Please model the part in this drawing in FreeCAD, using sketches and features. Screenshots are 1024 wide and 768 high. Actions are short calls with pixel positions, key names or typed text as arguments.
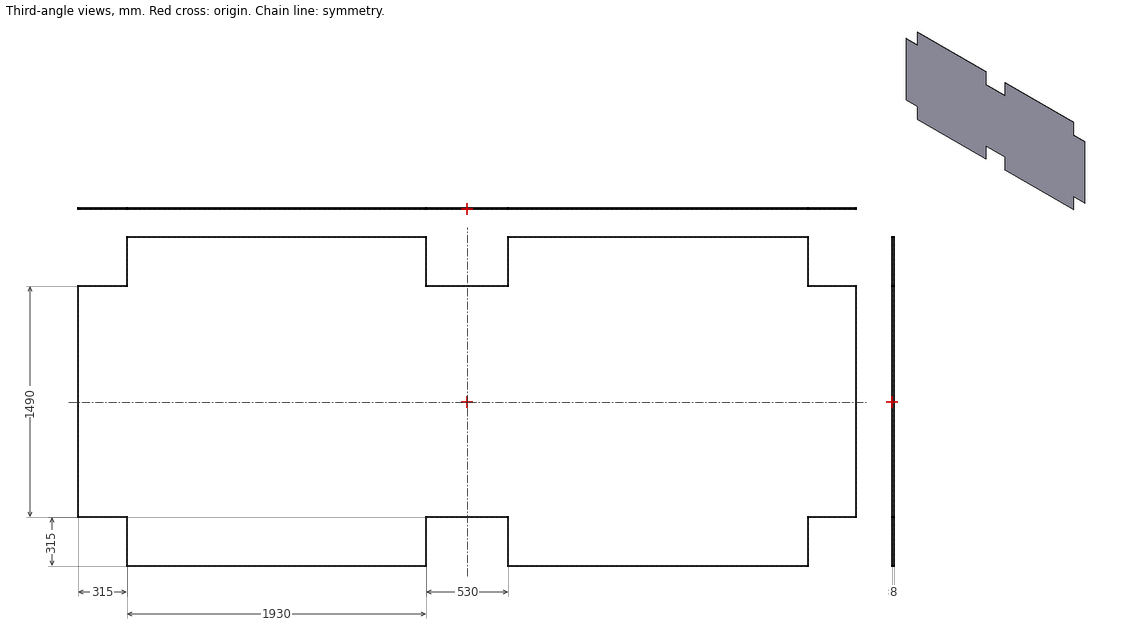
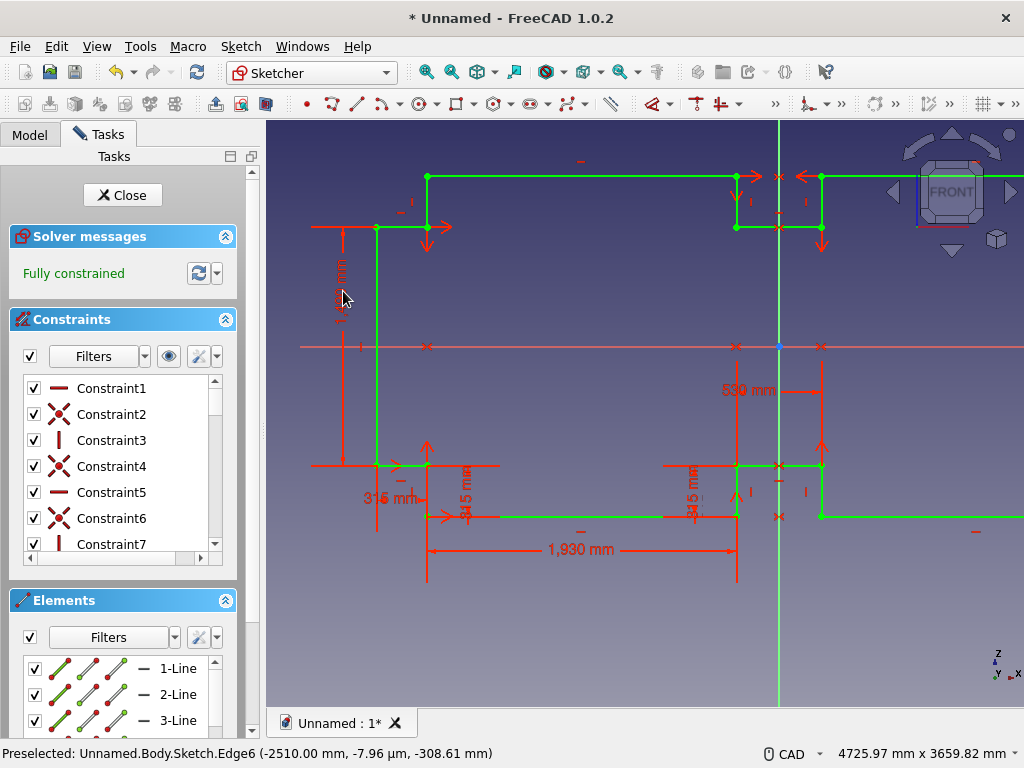
click(123, 195)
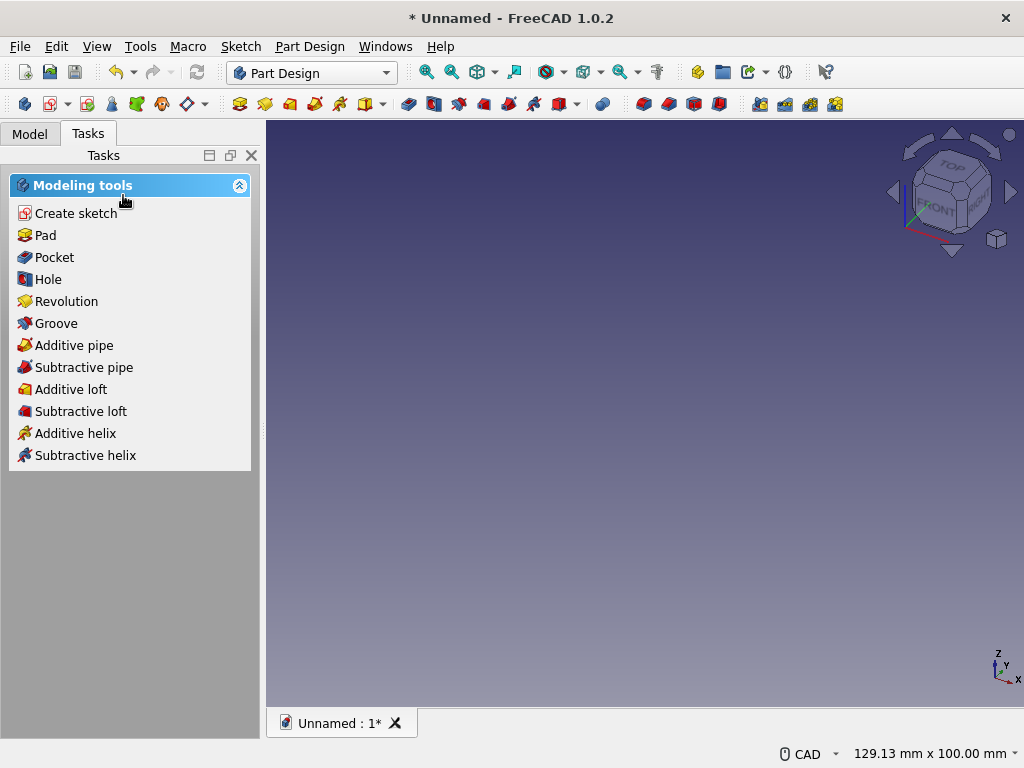
click(240, 104)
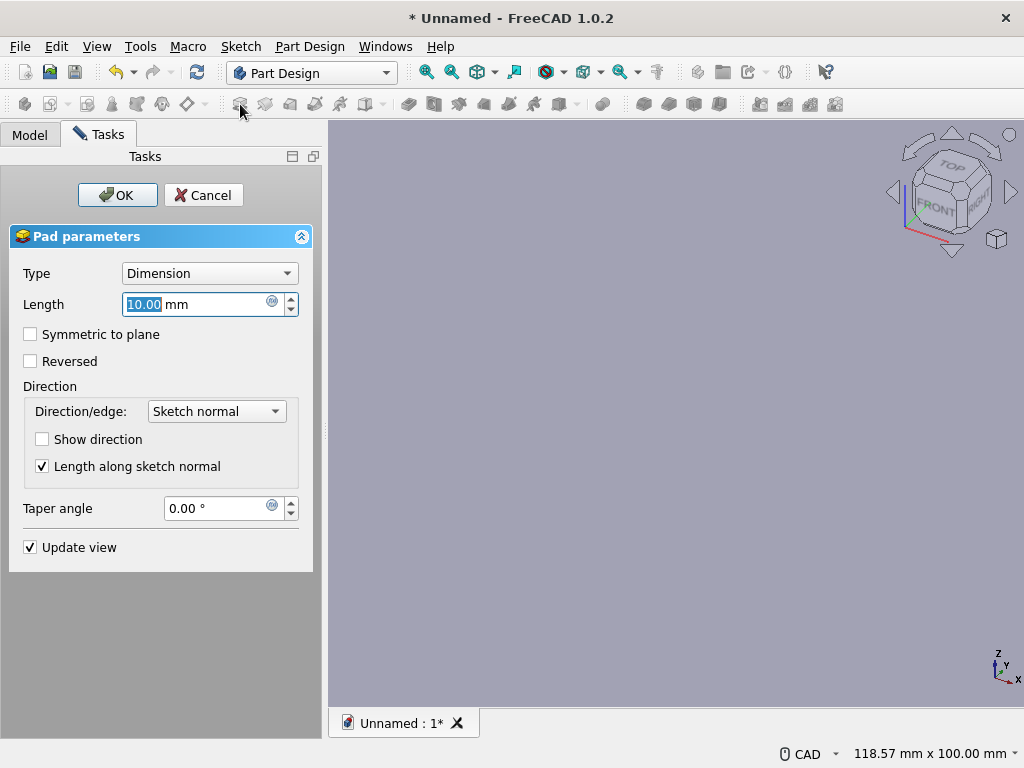
text(8)
key(Tab)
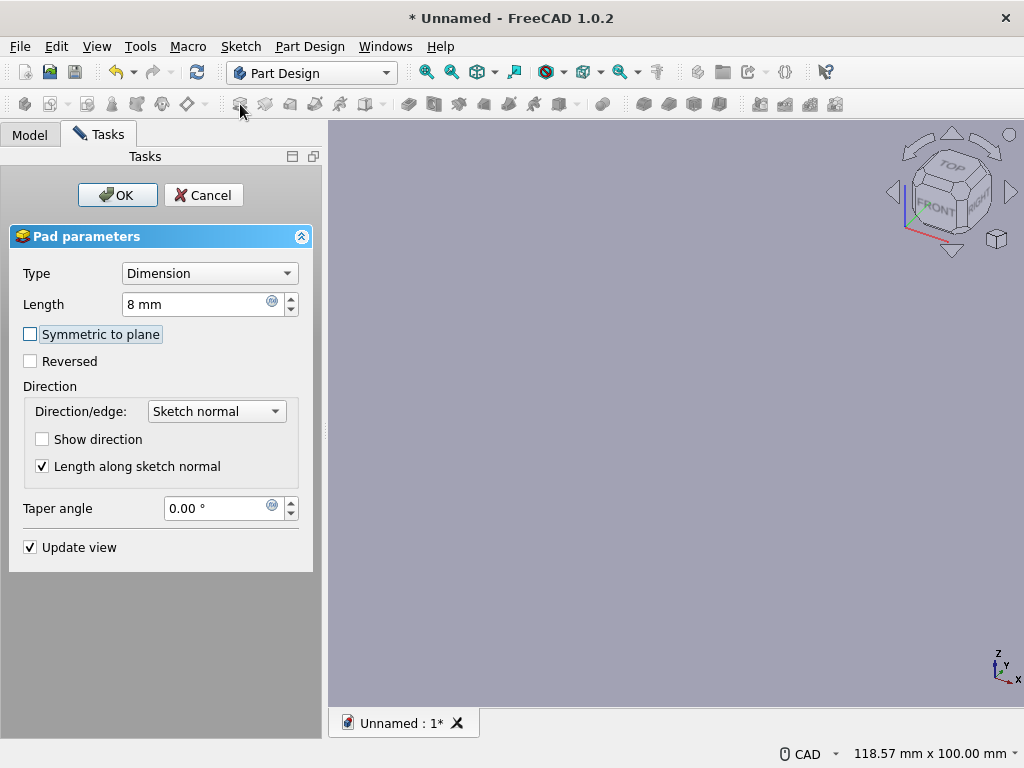
click(31, 361)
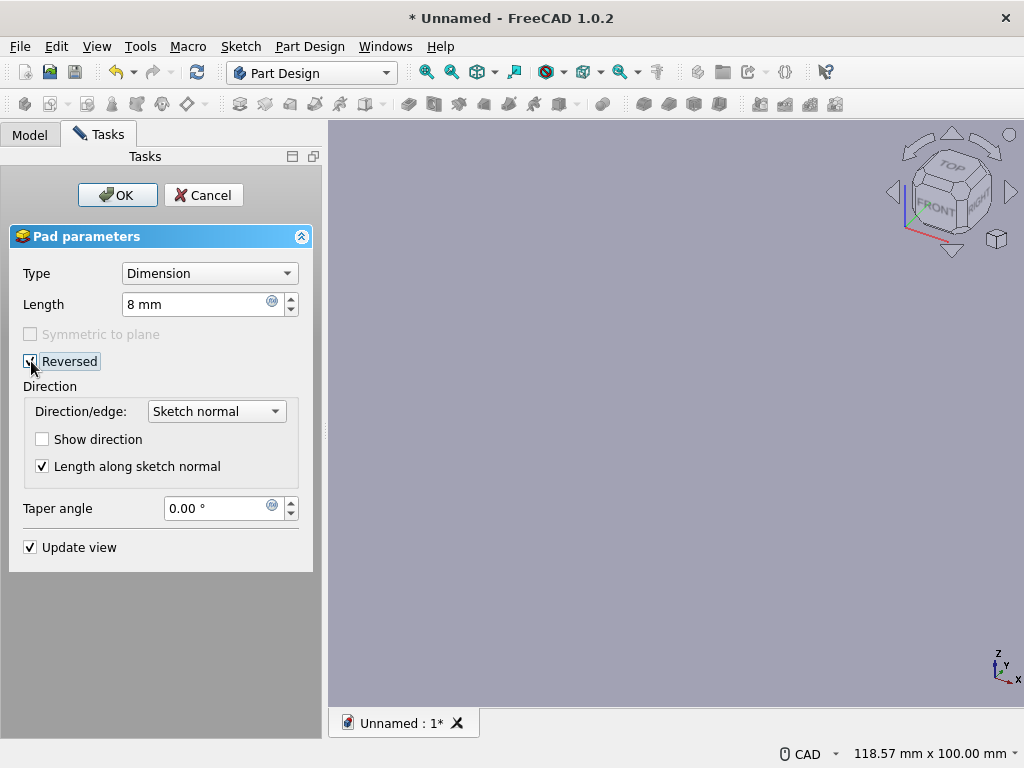
click(118, 195)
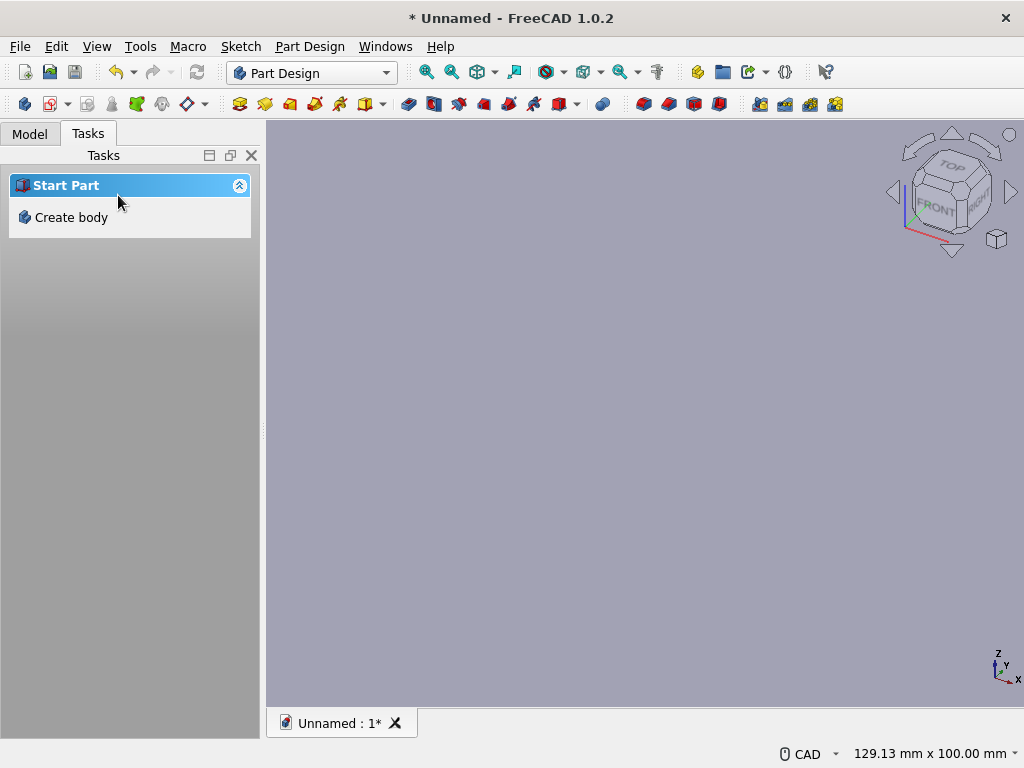
key(0)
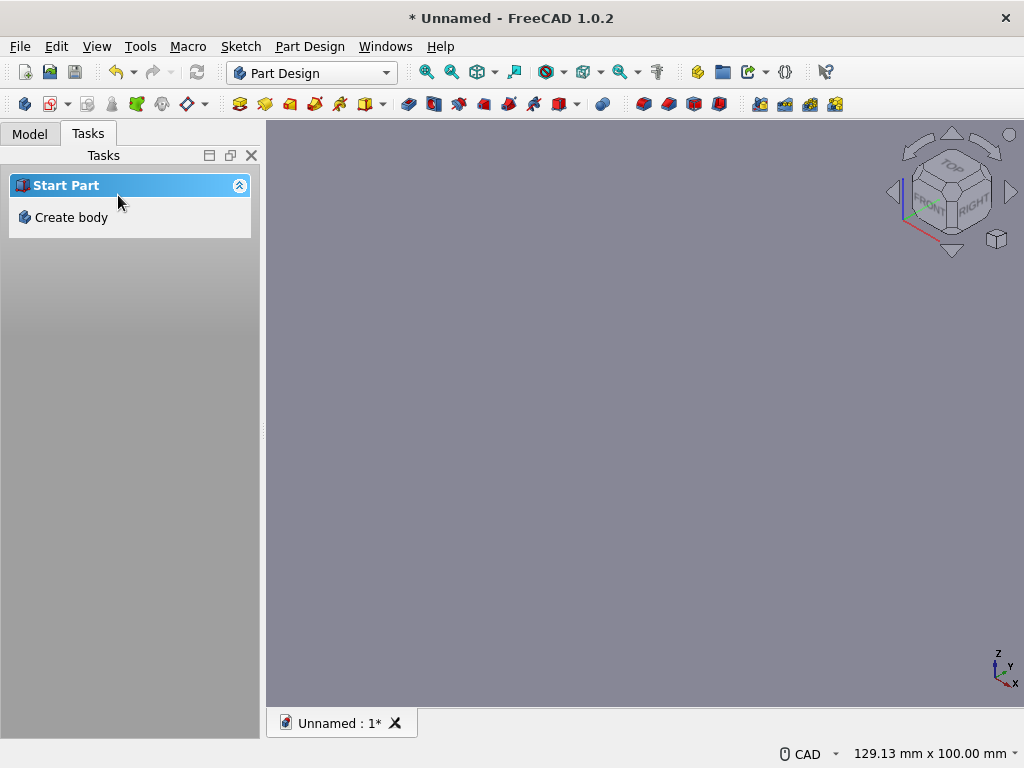
click(427, 72)